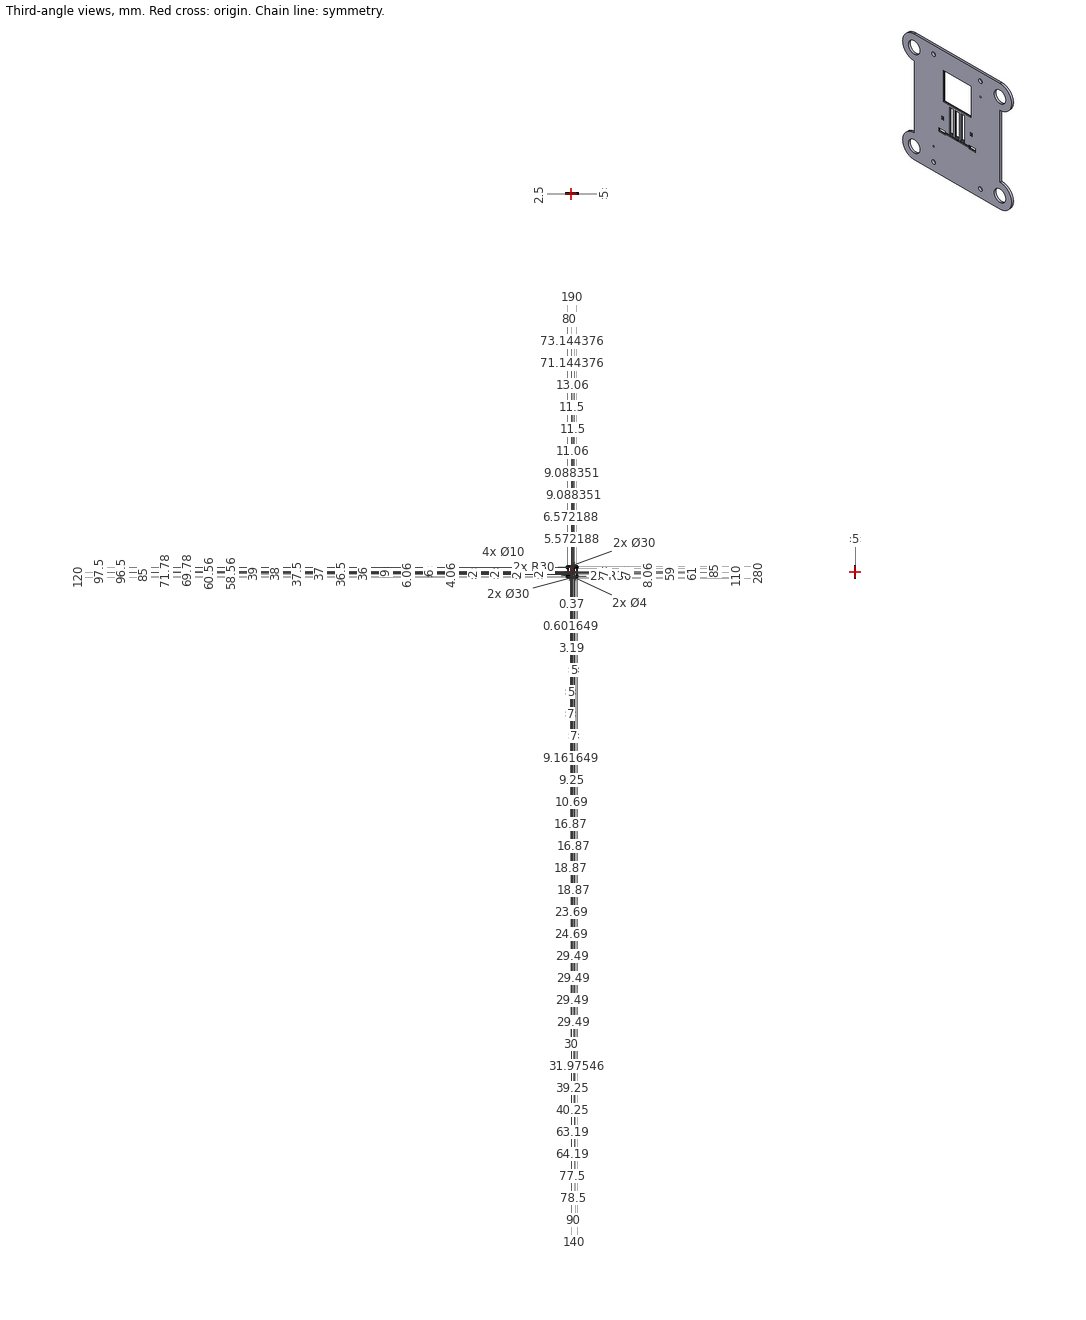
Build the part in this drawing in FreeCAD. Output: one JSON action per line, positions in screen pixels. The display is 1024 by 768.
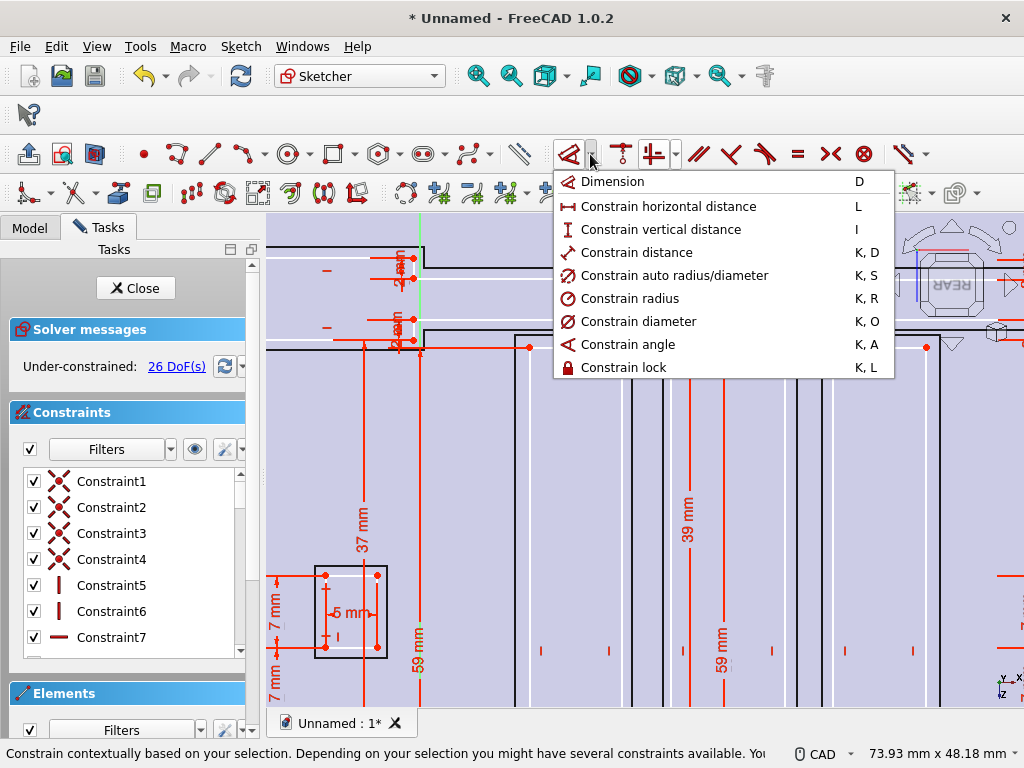
{"action": "left_click", "coordinate": [724, 230]}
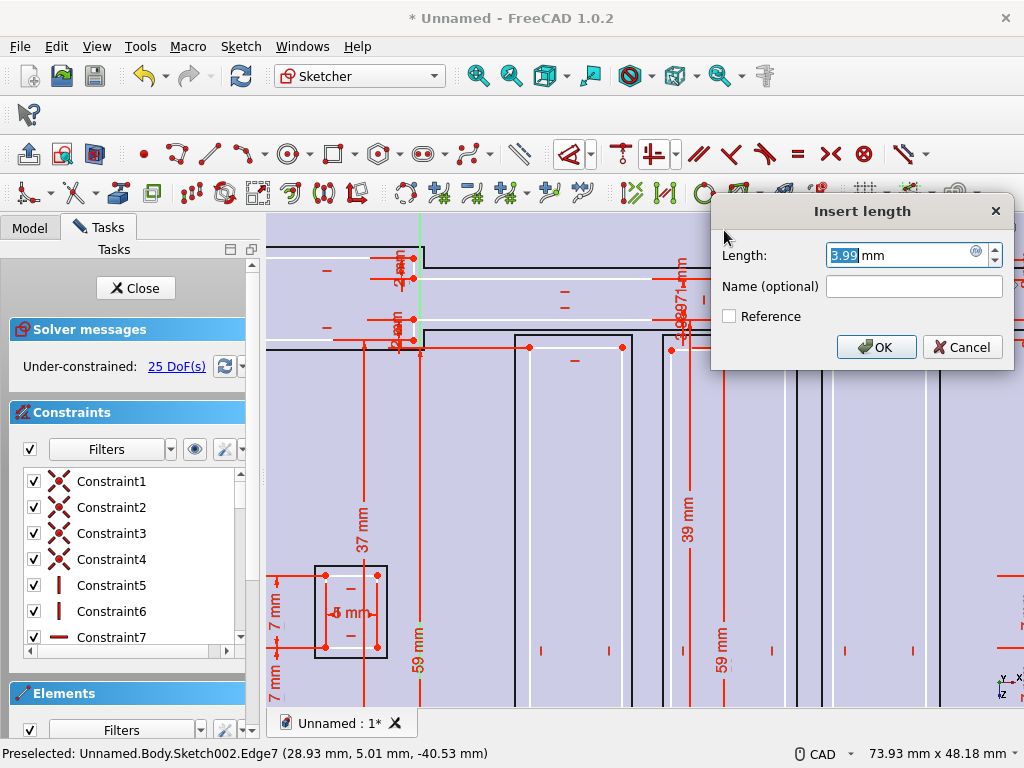
{"action": "type", "text": "4.06"}
{"action": "key", "text": "Return"}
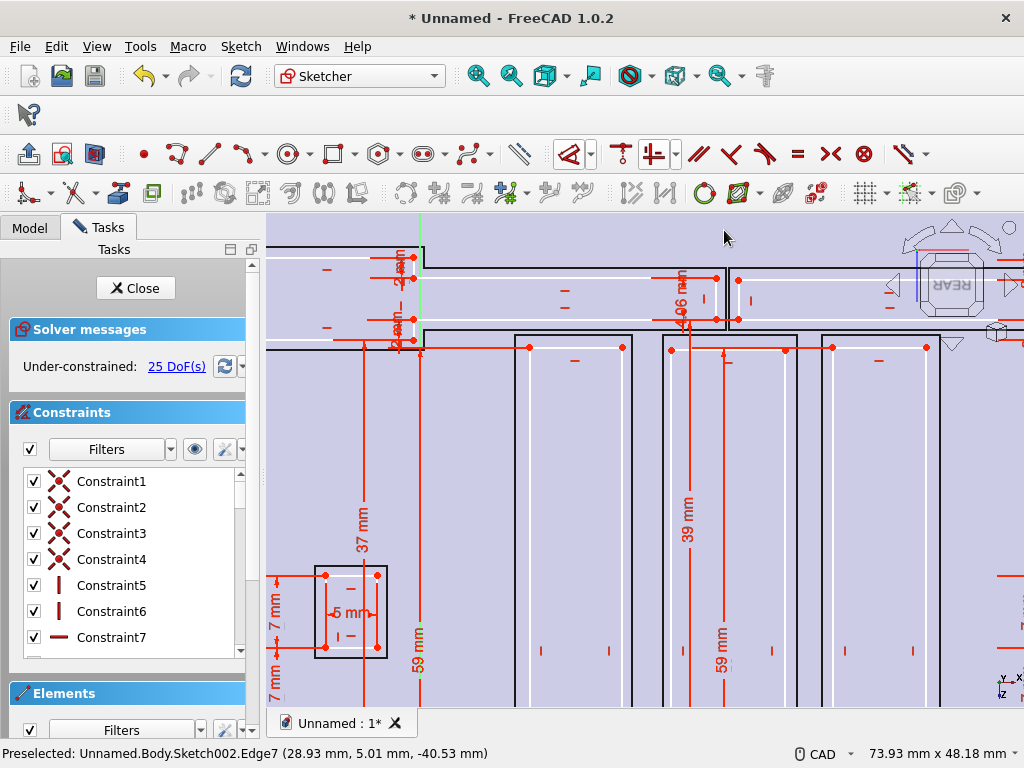
{"action": "scroll", "coordinate": [538, 328], "scroll_direction": "down", "scroll_amount": 8}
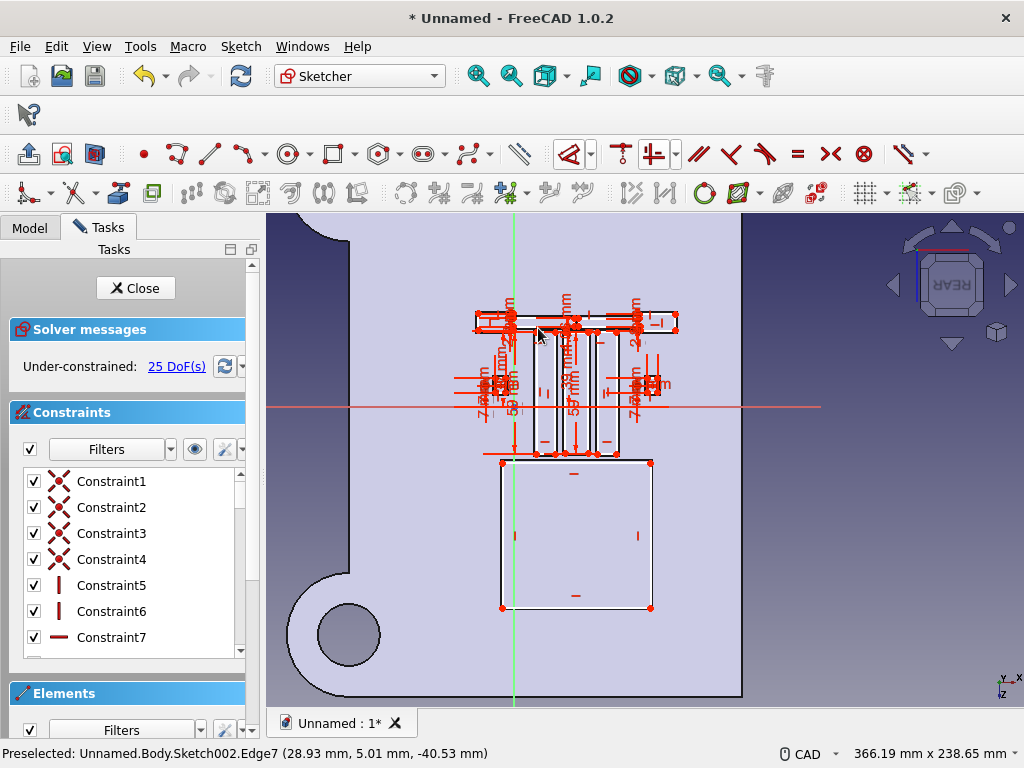
{"action": "scroll", "coordinate": [675, 326], "scroll_direction": "up", "scroll_amount": 6}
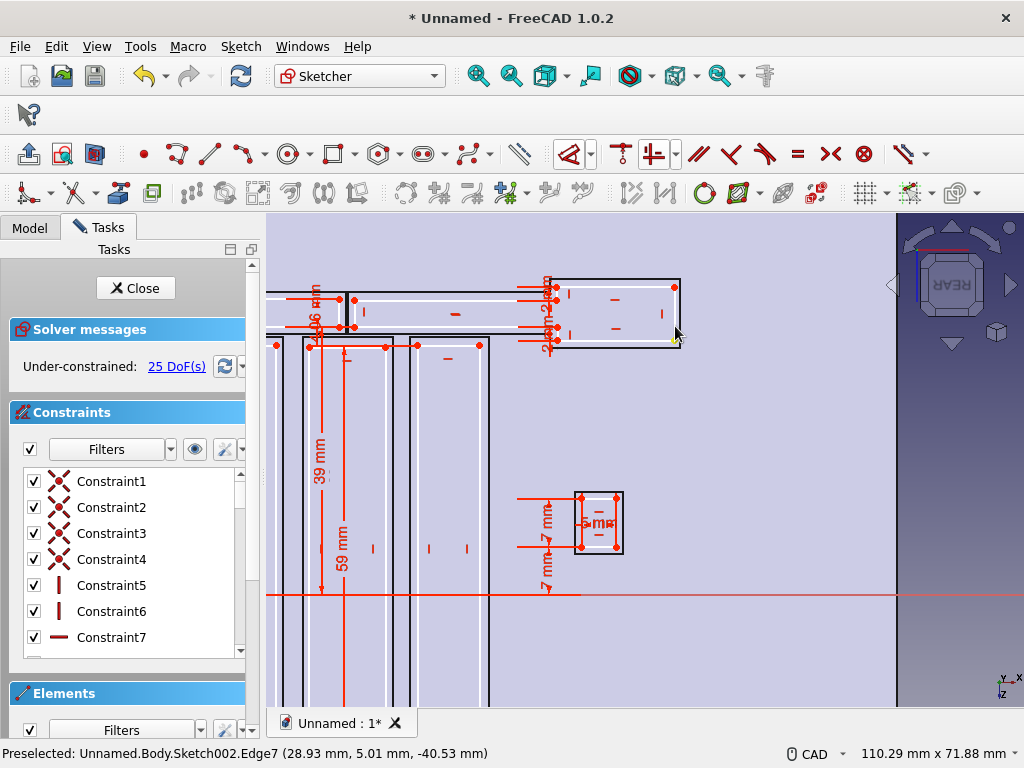
{"action": "left_click", "coordinate": [675, 325]}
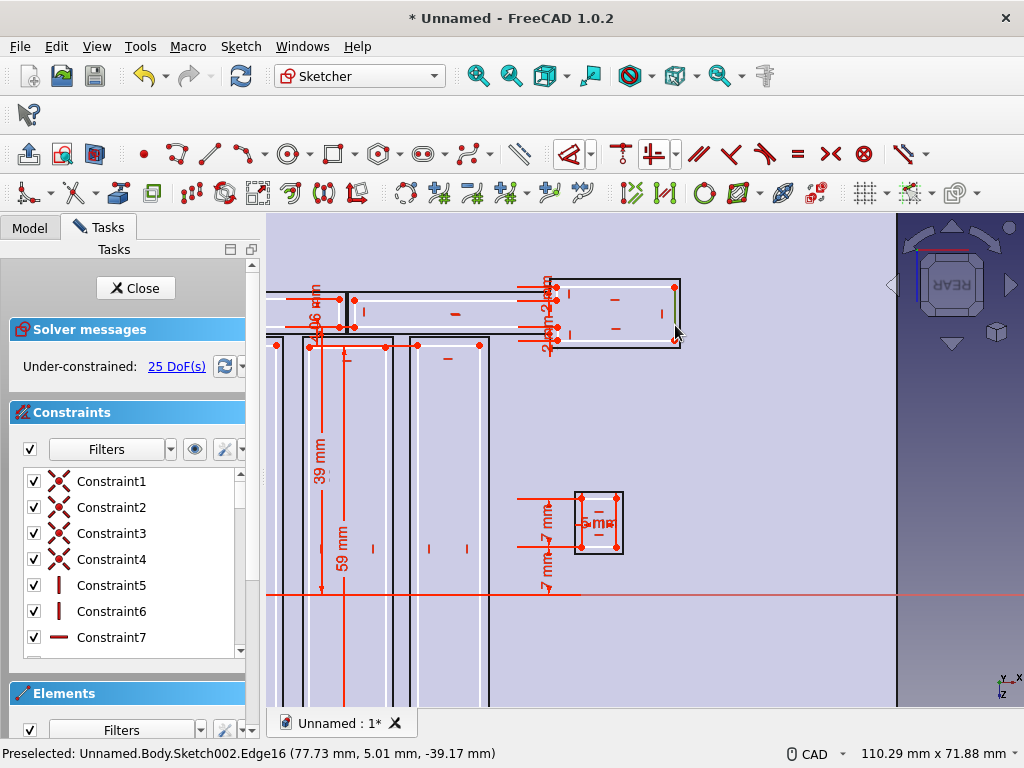
{"action": "left_click", "coordinate": [590, 154]}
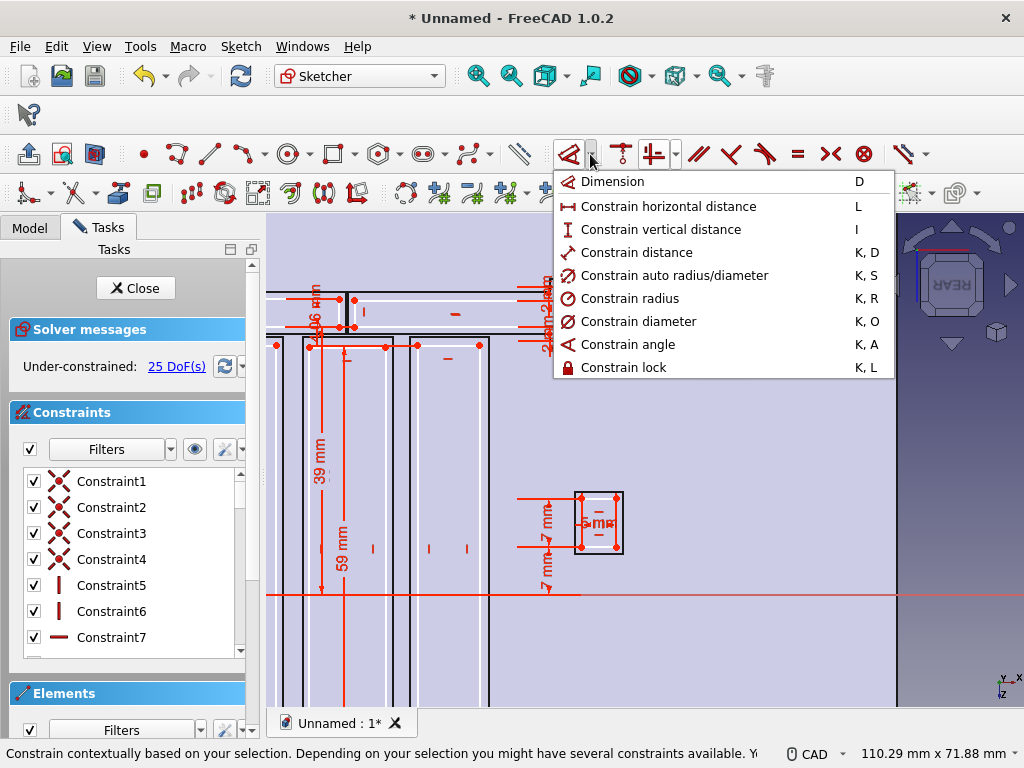
{"action": "left_click", "coordinate": [724, 230]}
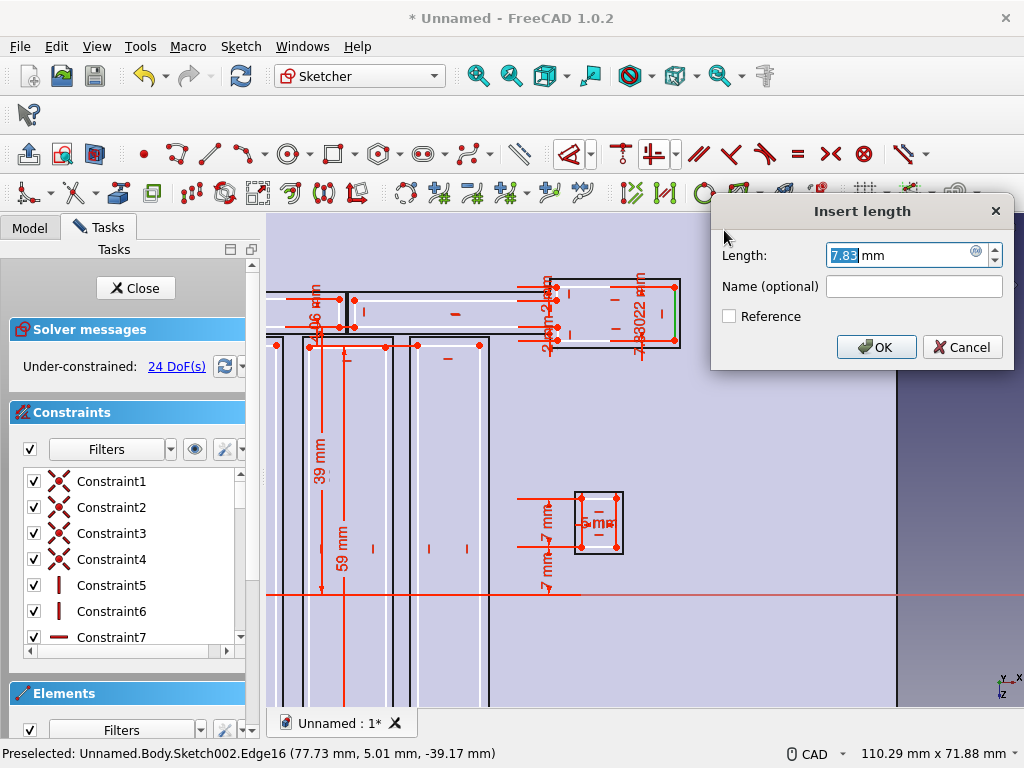
{"action": "type", "text": "8.06"}
{"action": "key", "text": "Return"}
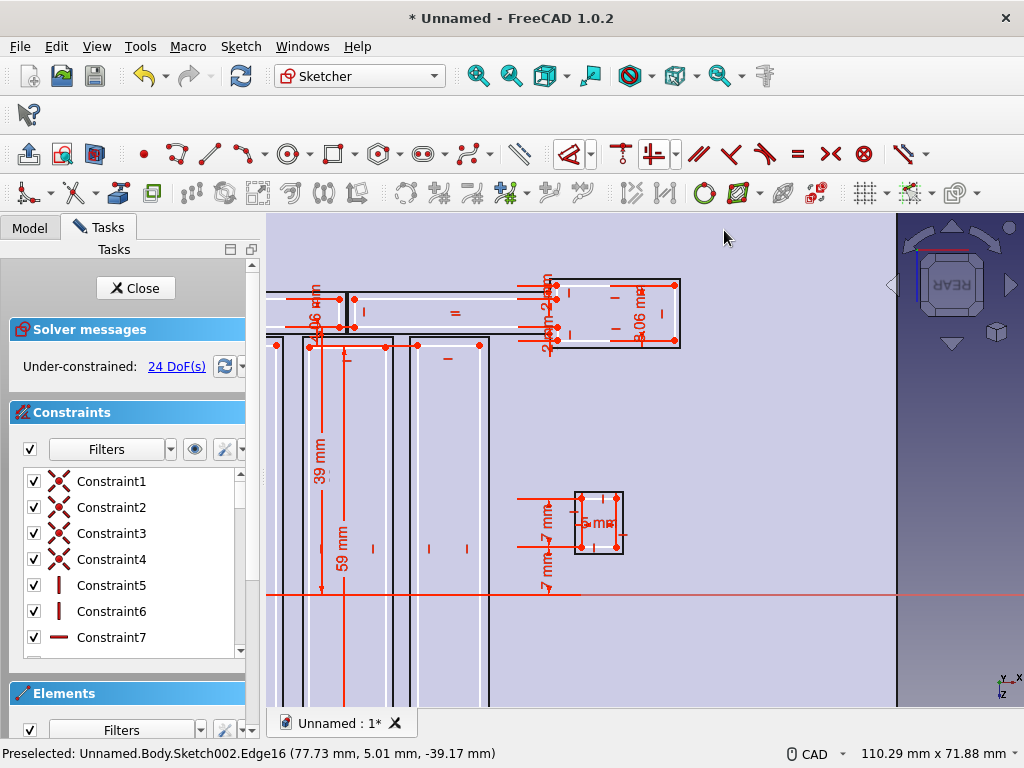
{"action": "left_click", "coordinate": [309, 468]}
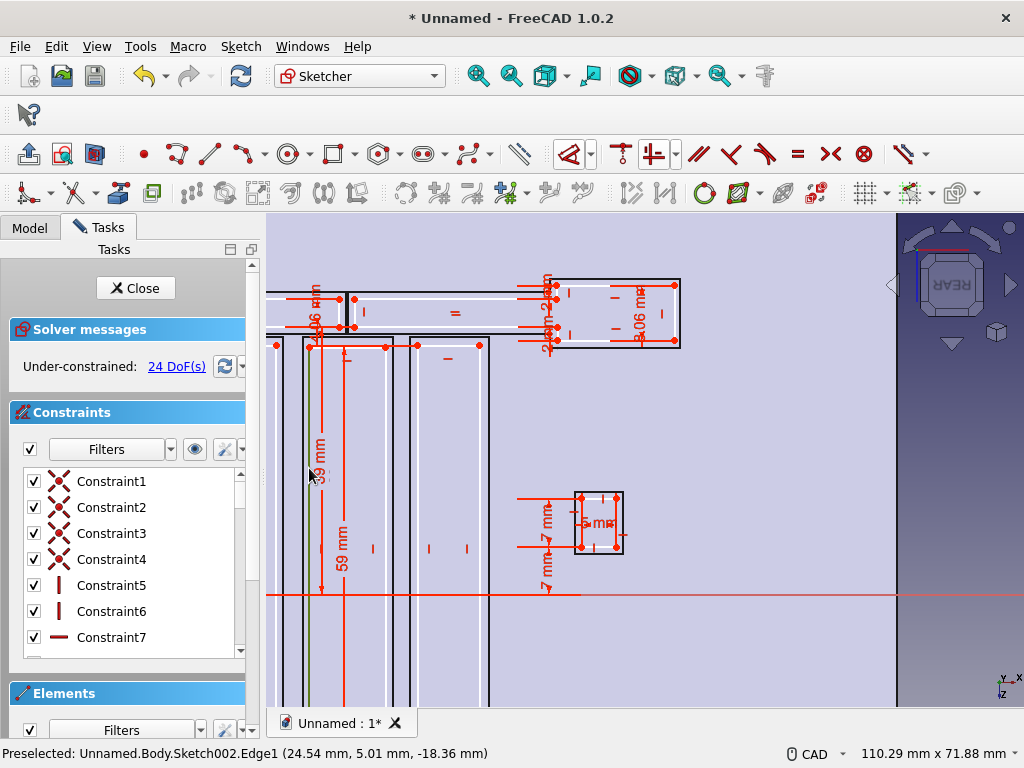
{"action": "left_click", "coordinate": [590, 154]}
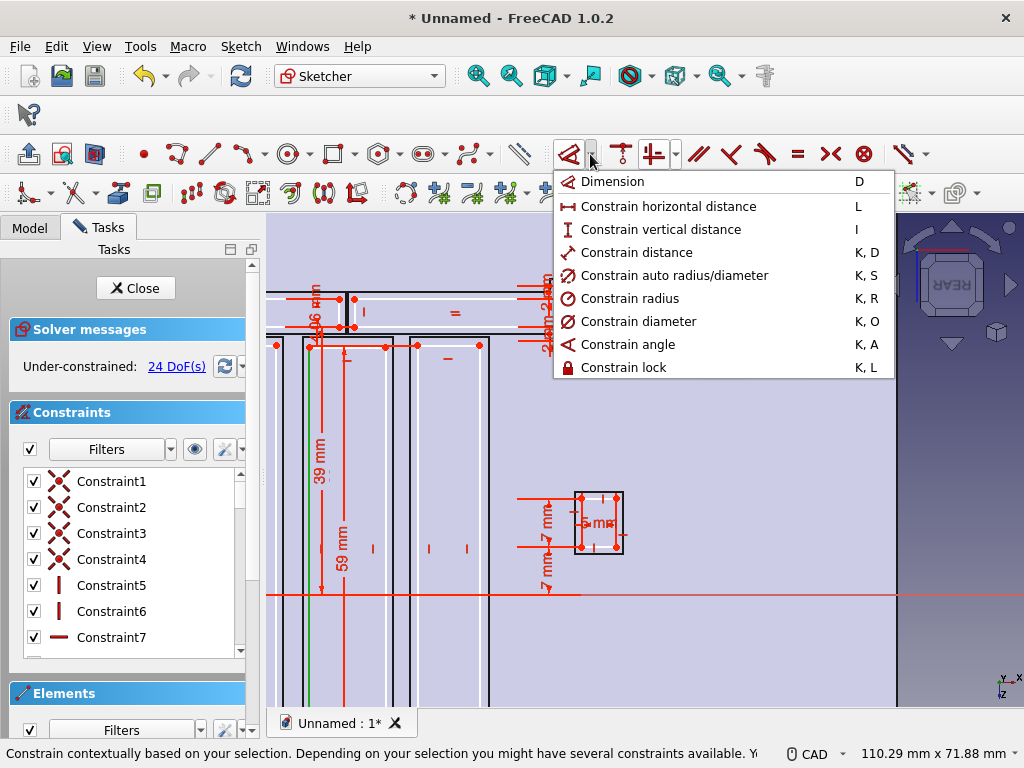
{"action": "left_click", "coordinate": [724, 230]}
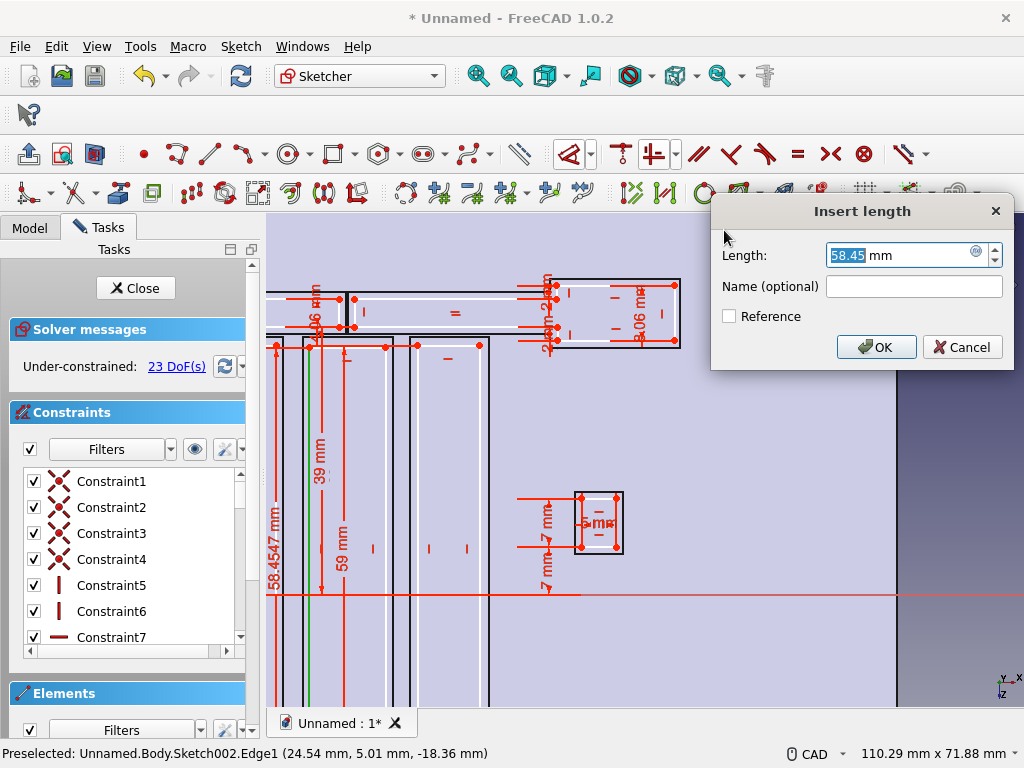
{"action": "type", "text": "58.56"}
{"action": "key", "text": "Return"}